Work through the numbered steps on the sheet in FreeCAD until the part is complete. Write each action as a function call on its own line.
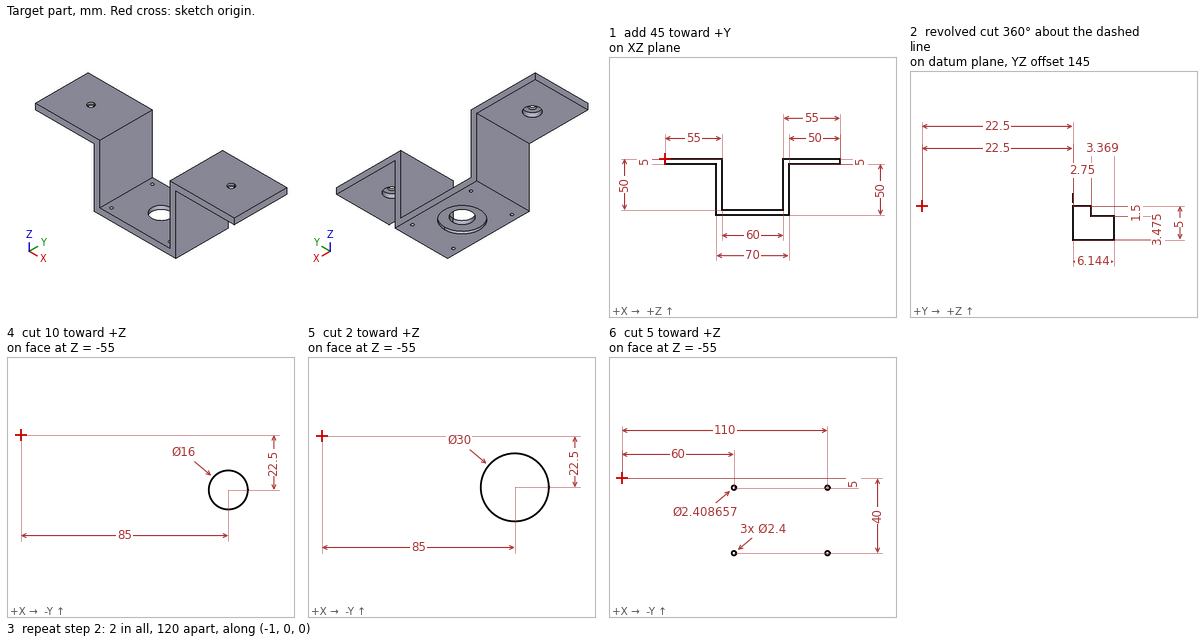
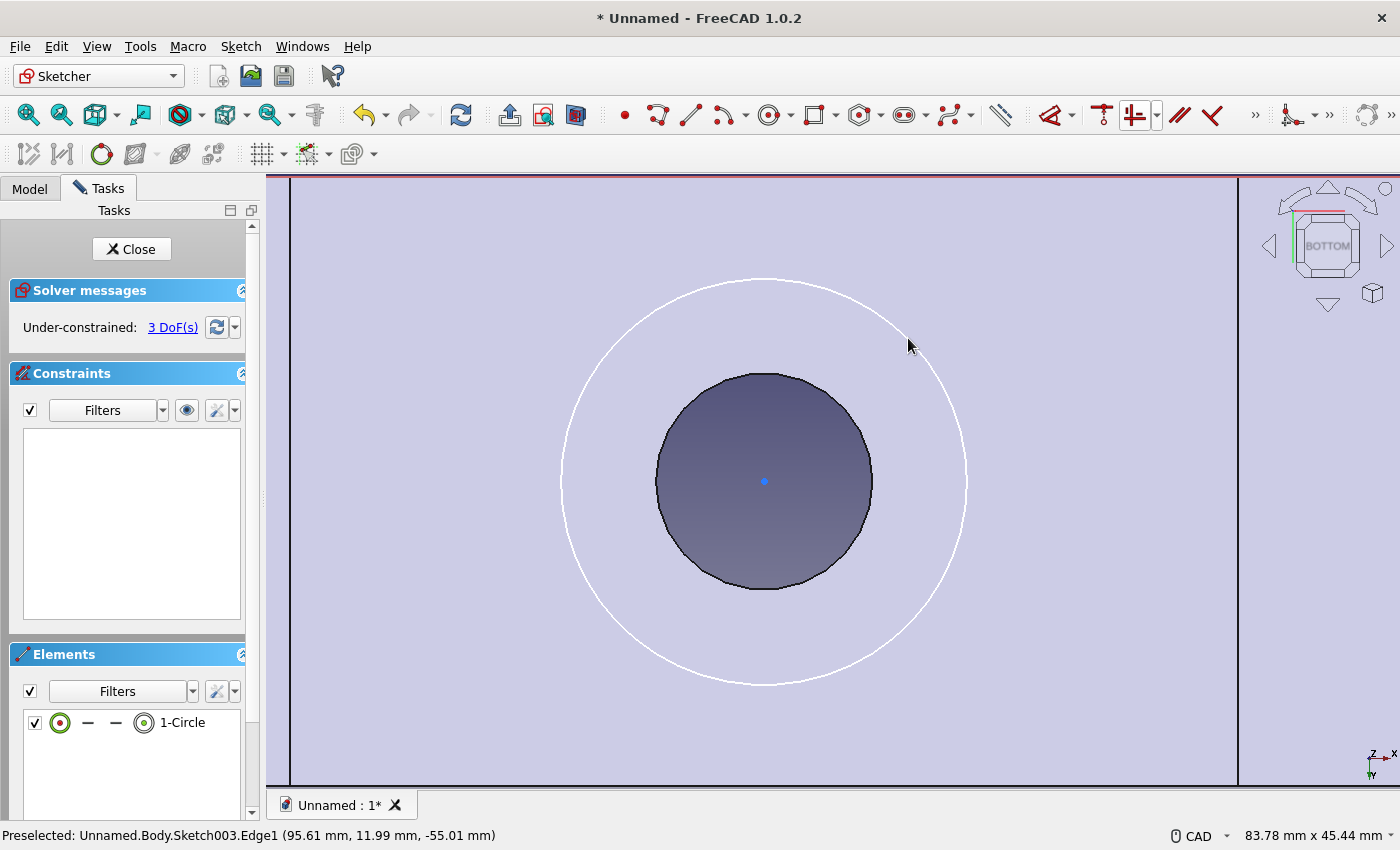
click(1050, 116)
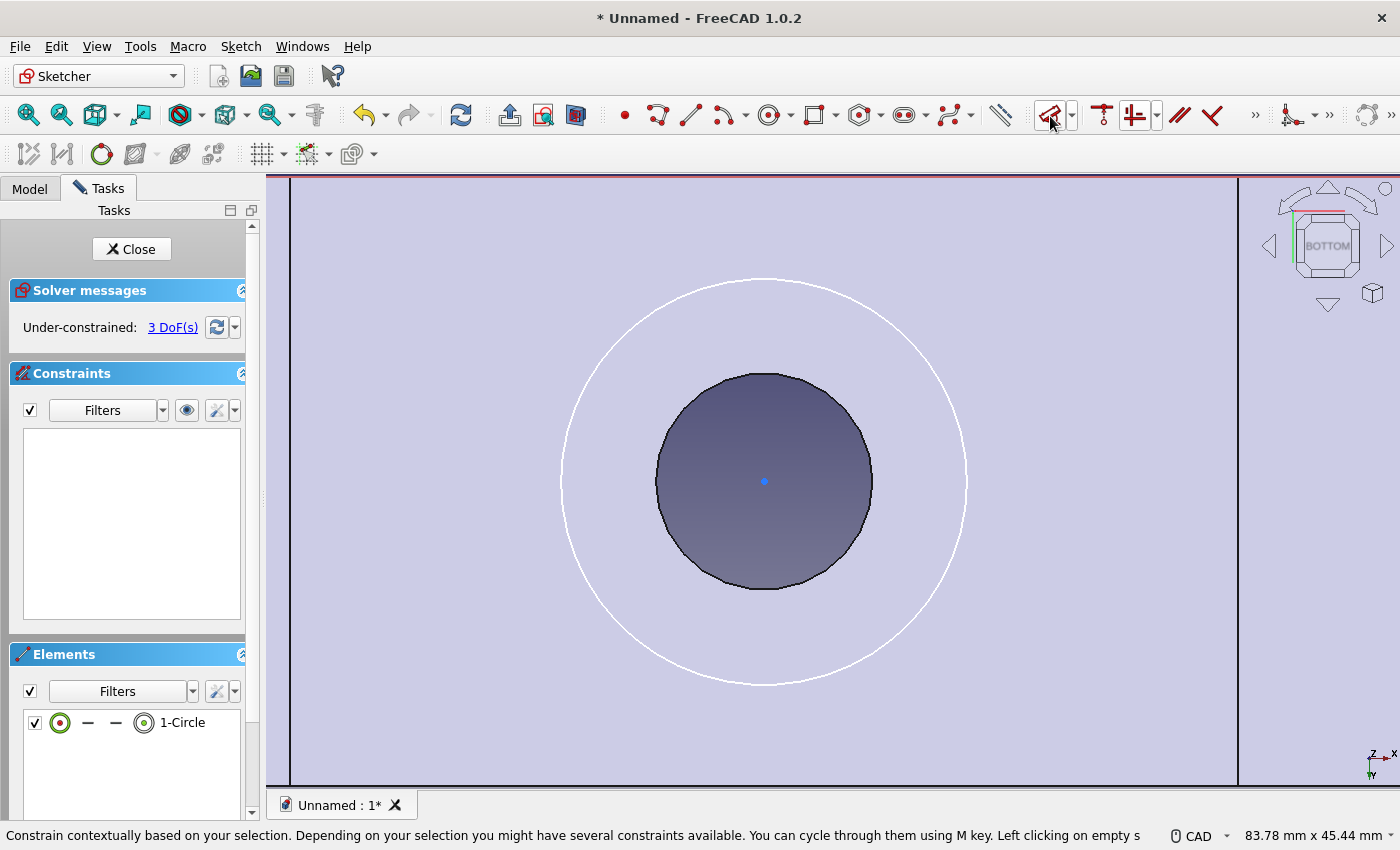
click(907, 338)
click(930, 315)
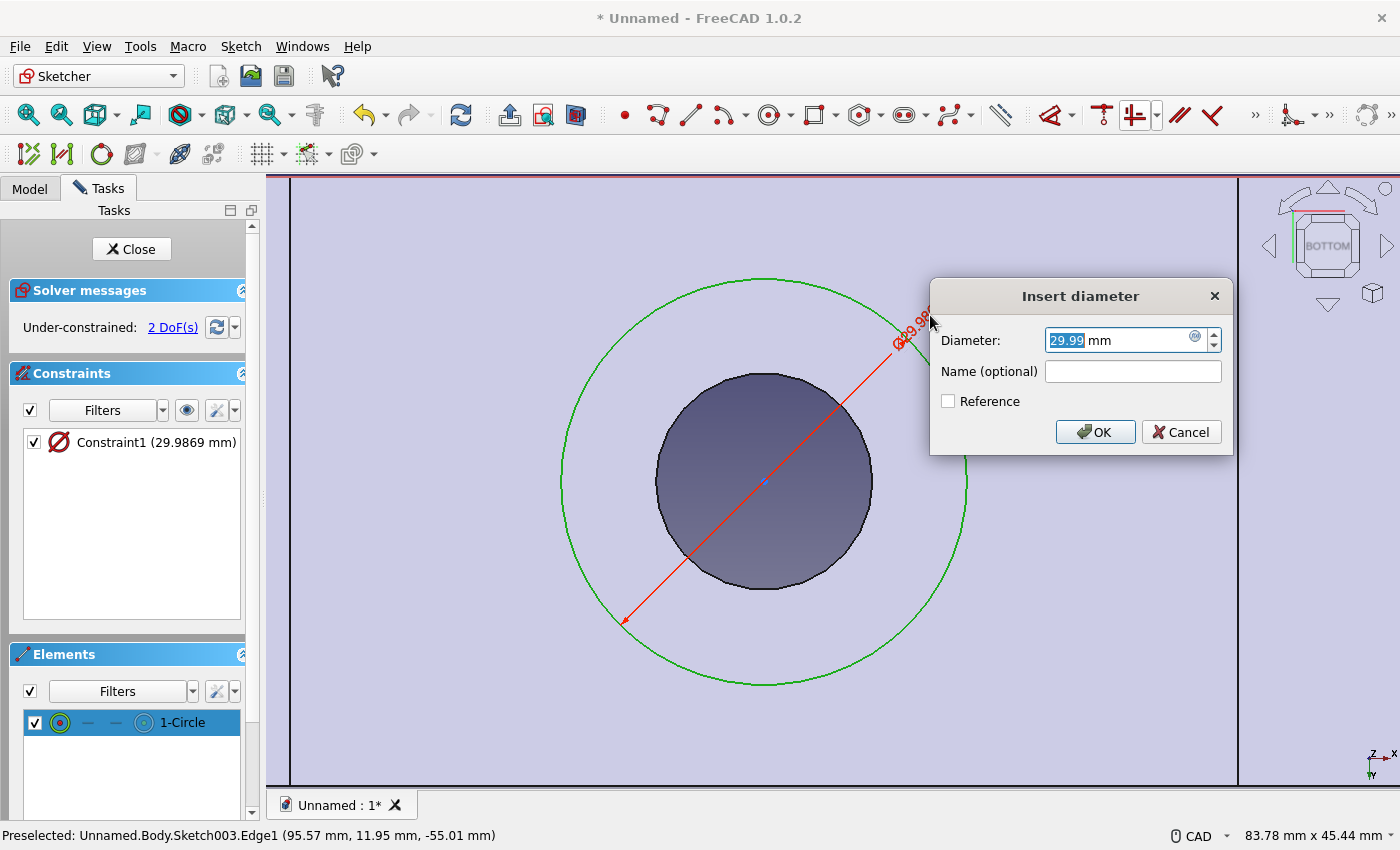
text(30)
key(Return)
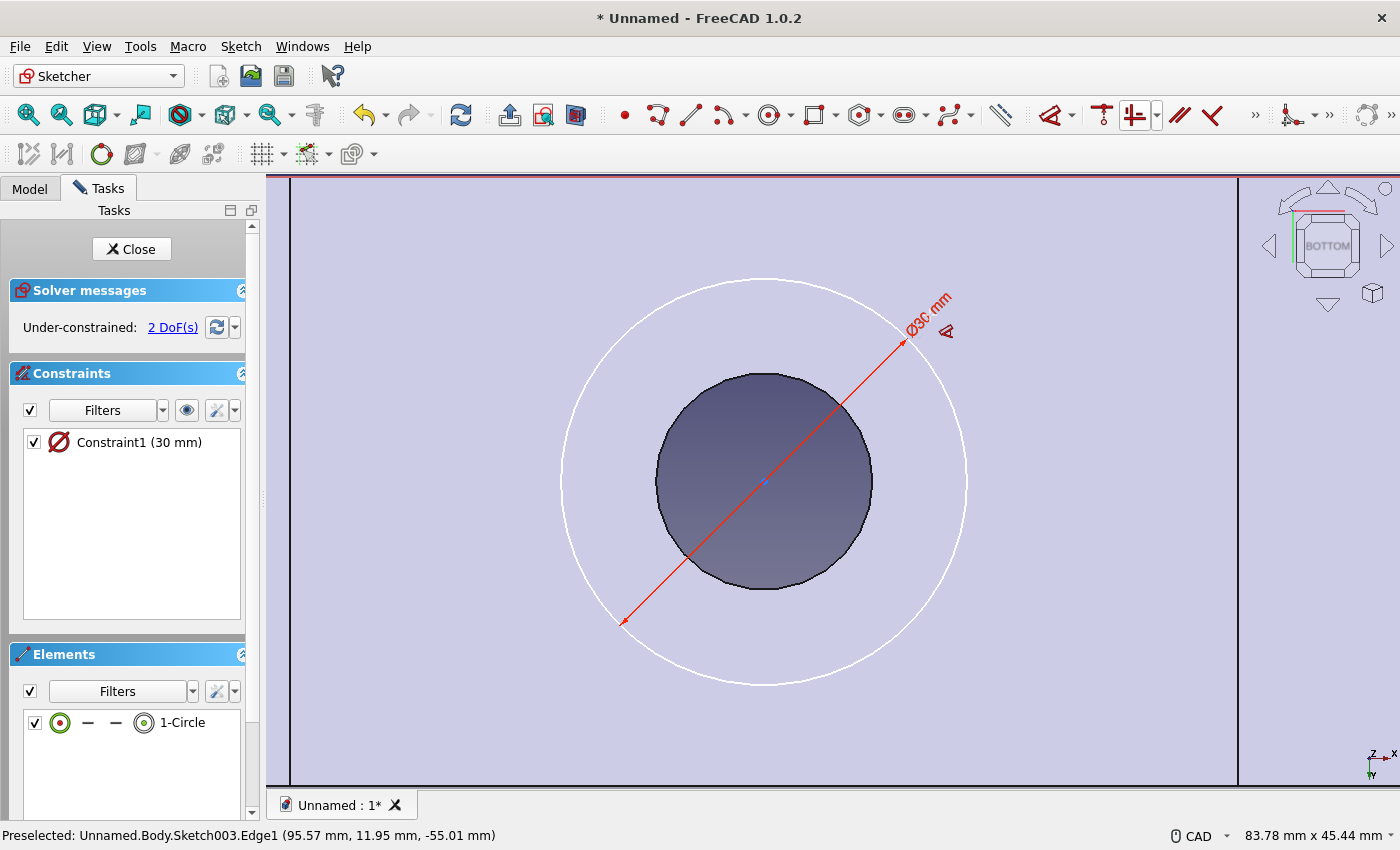
click(764, 482)
click(529, 516)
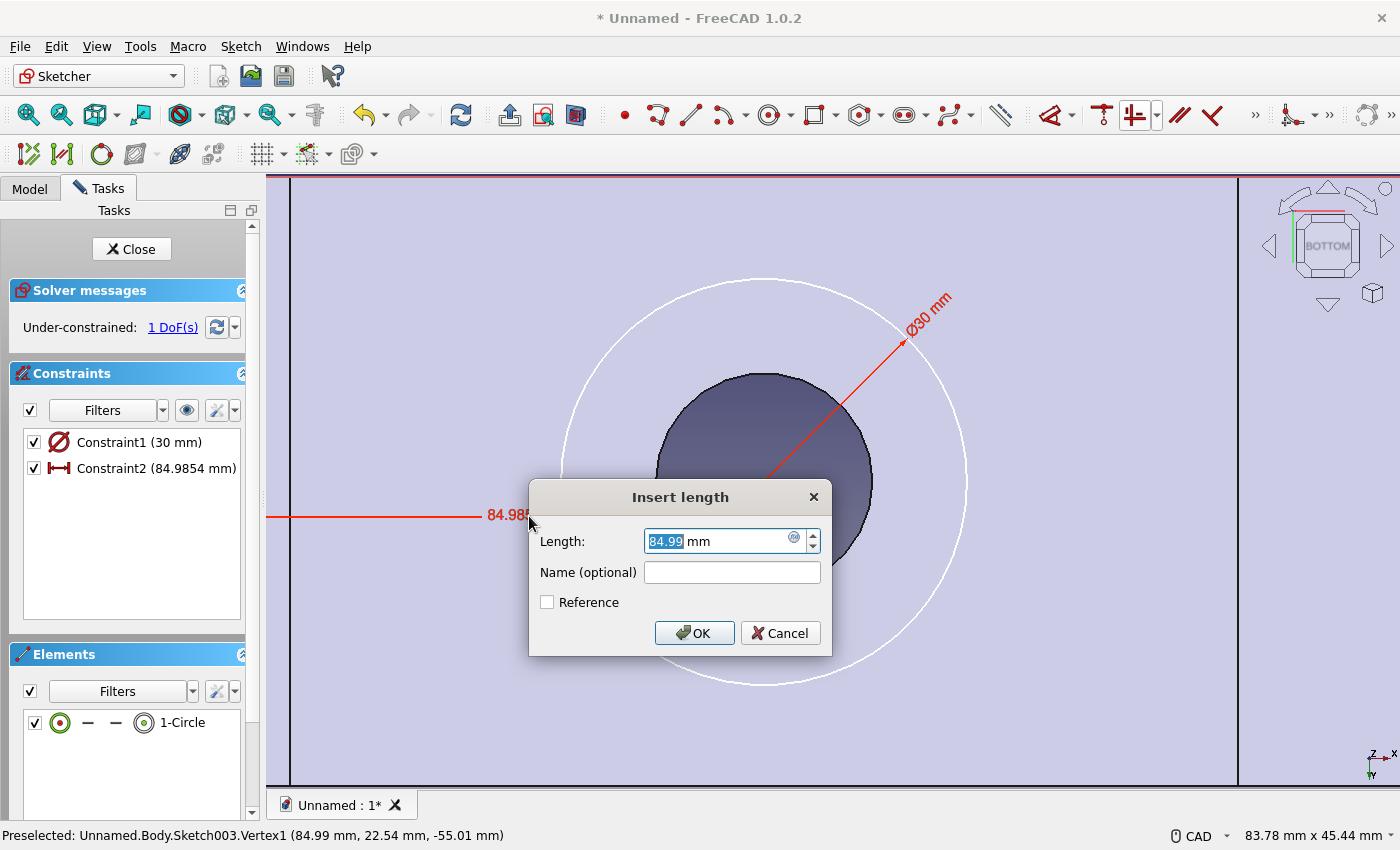
text(85)
key(Return)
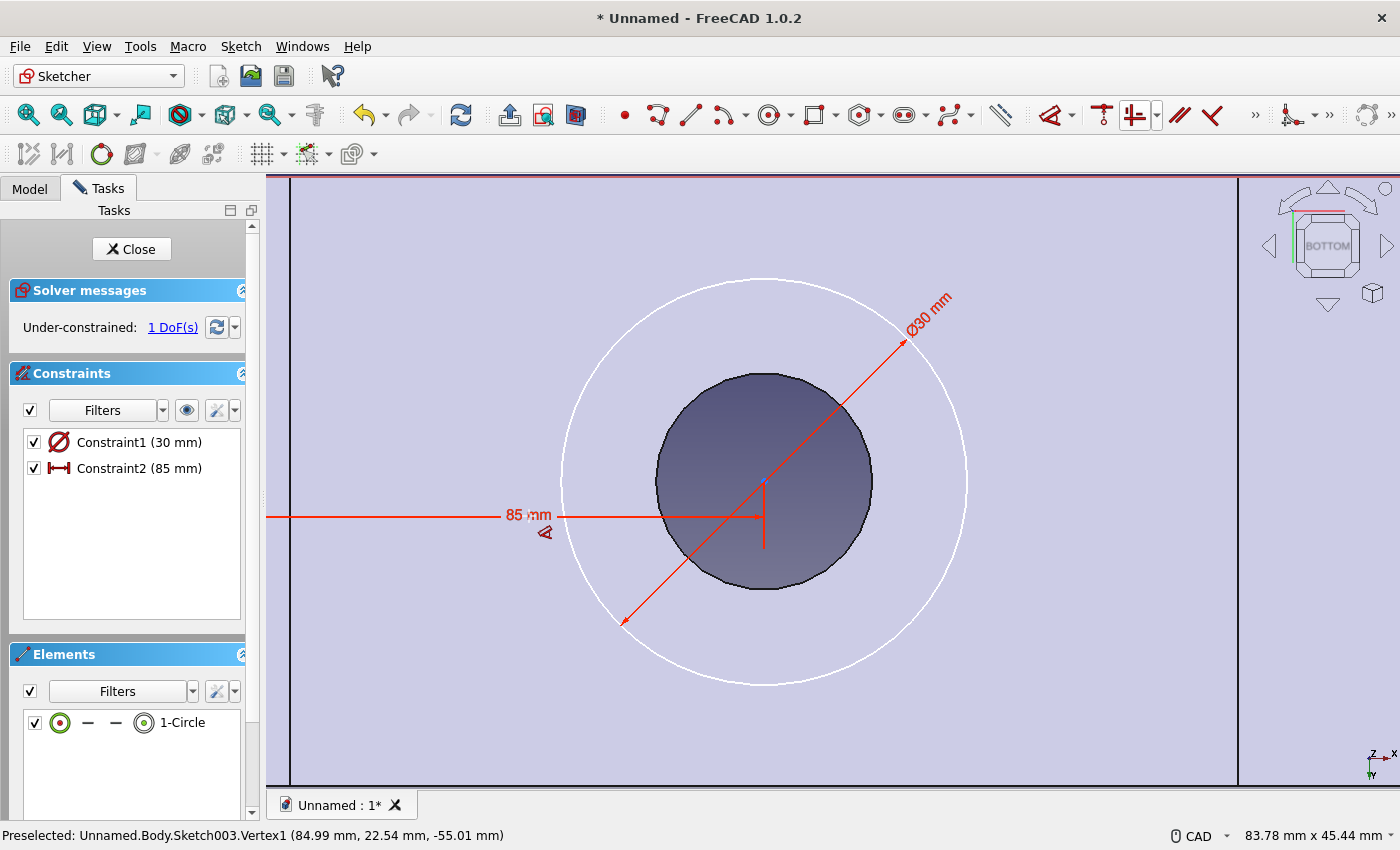
click(764, 482)
click(798, 342)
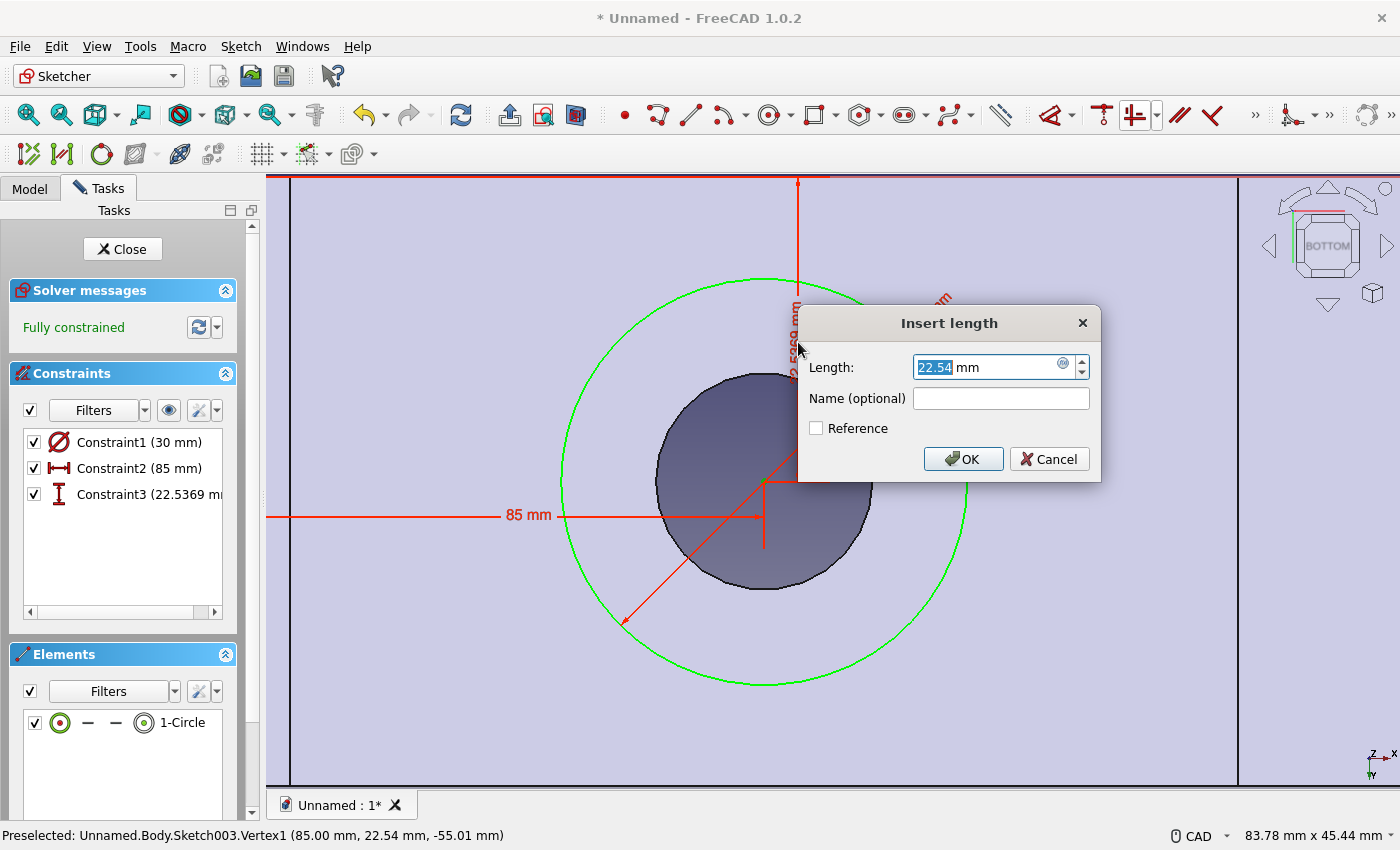
text(22.5)
key(Return)
key(Escape)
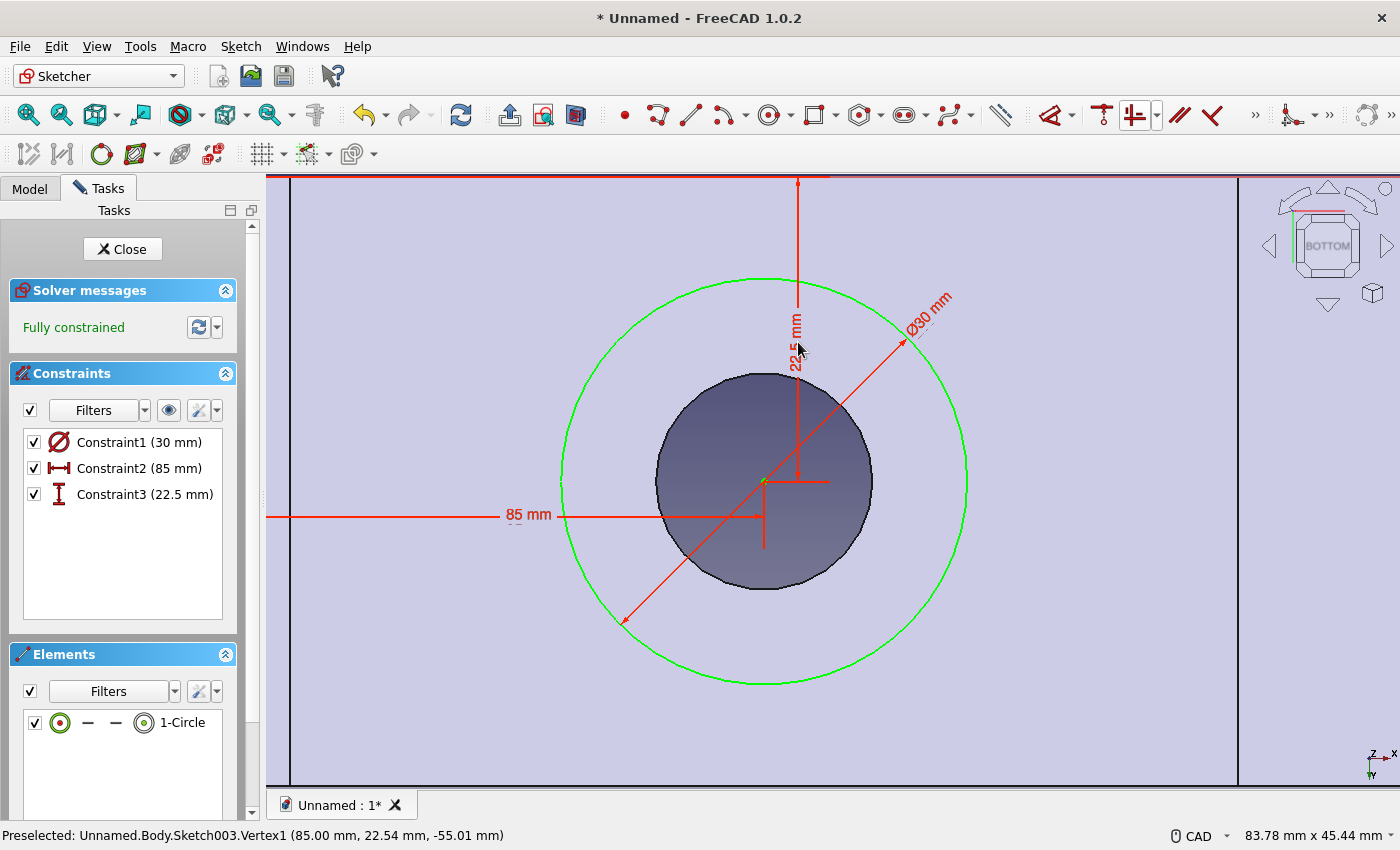
click(123, 249)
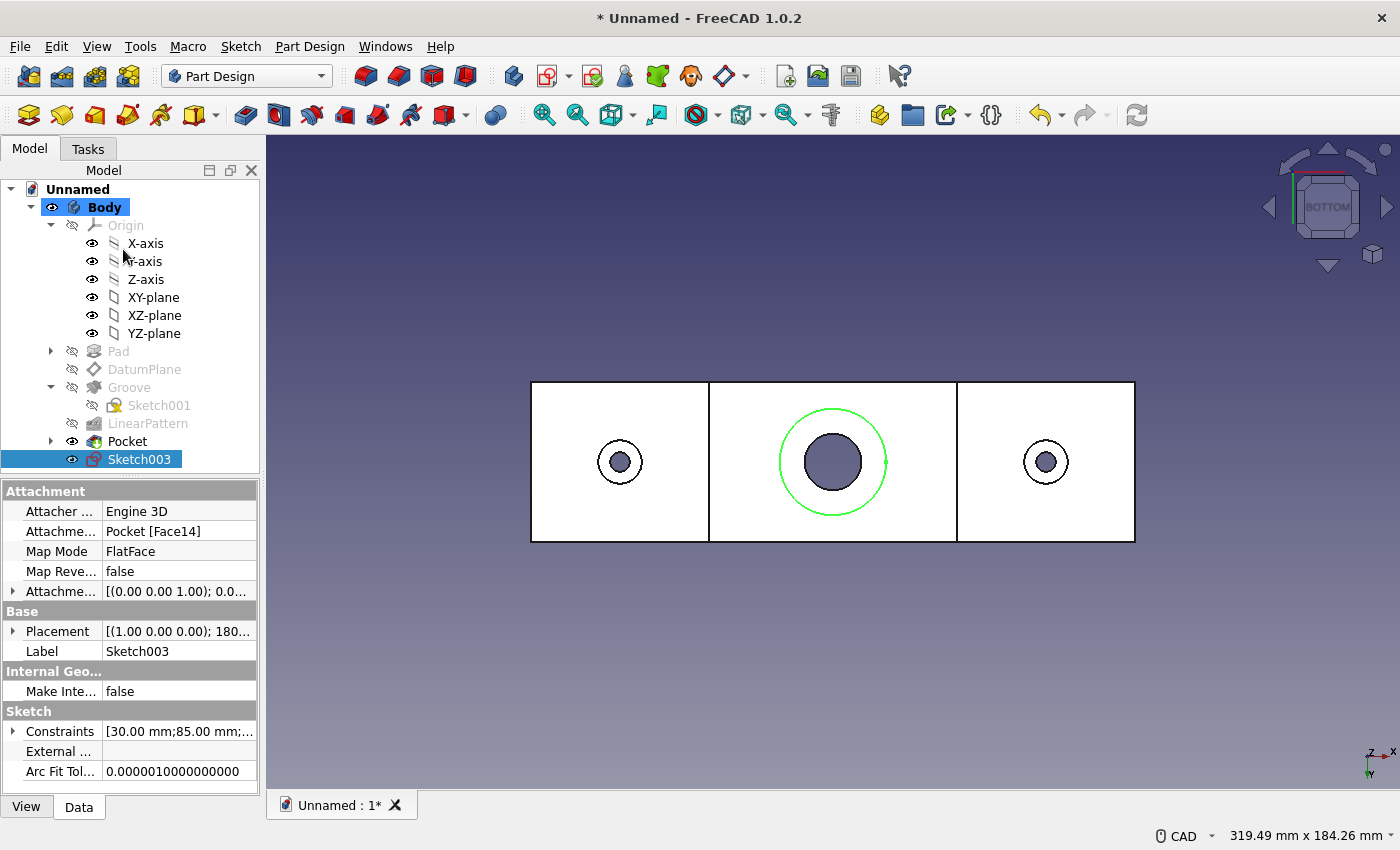
click(246, 116)